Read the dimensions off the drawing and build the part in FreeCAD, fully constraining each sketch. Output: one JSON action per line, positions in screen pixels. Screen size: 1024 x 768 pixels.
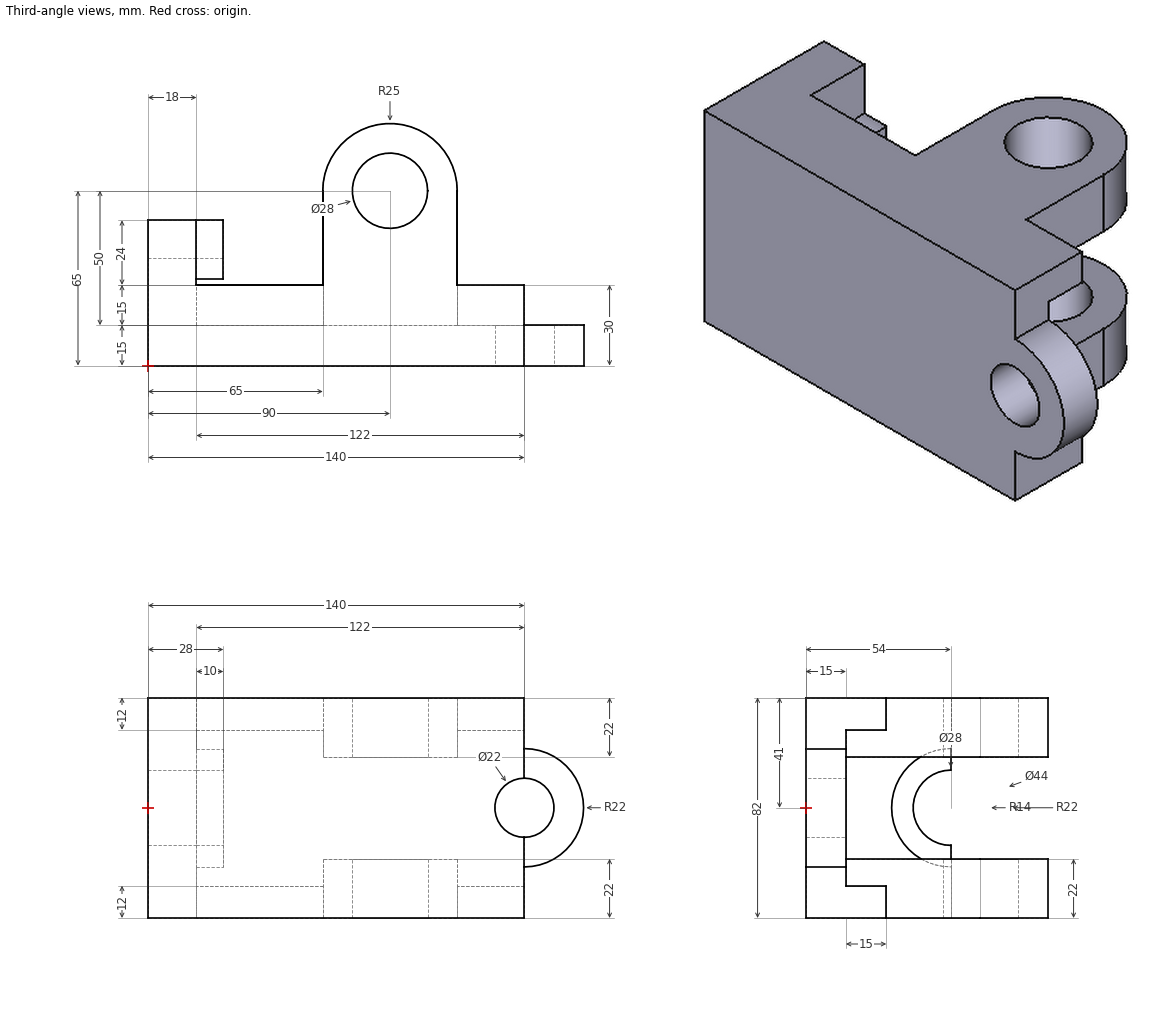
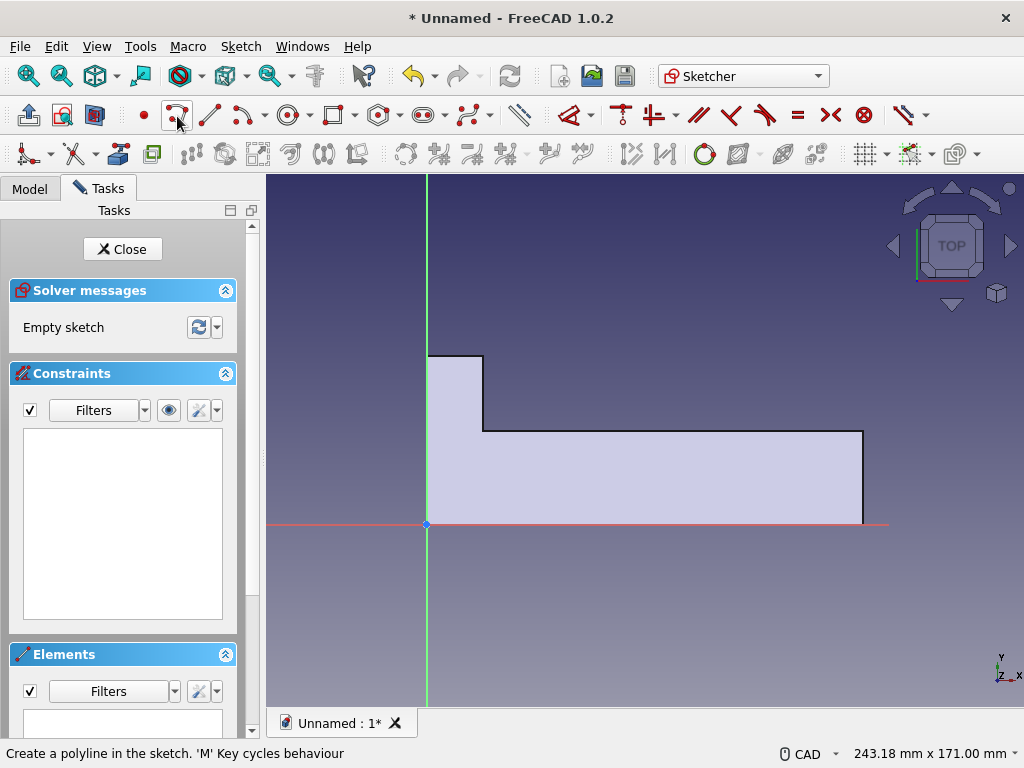
{"action": "left_click", "coordinate": [629, 322]}
{"action": "left_click", "coordinate": [629, 478]}
{"action": "left_click", "coordinate": [785, 478]}
{"action": "left_click", "coordinate": [785, 322]}
{"action": "right_click", "coordinate": [785, 322]}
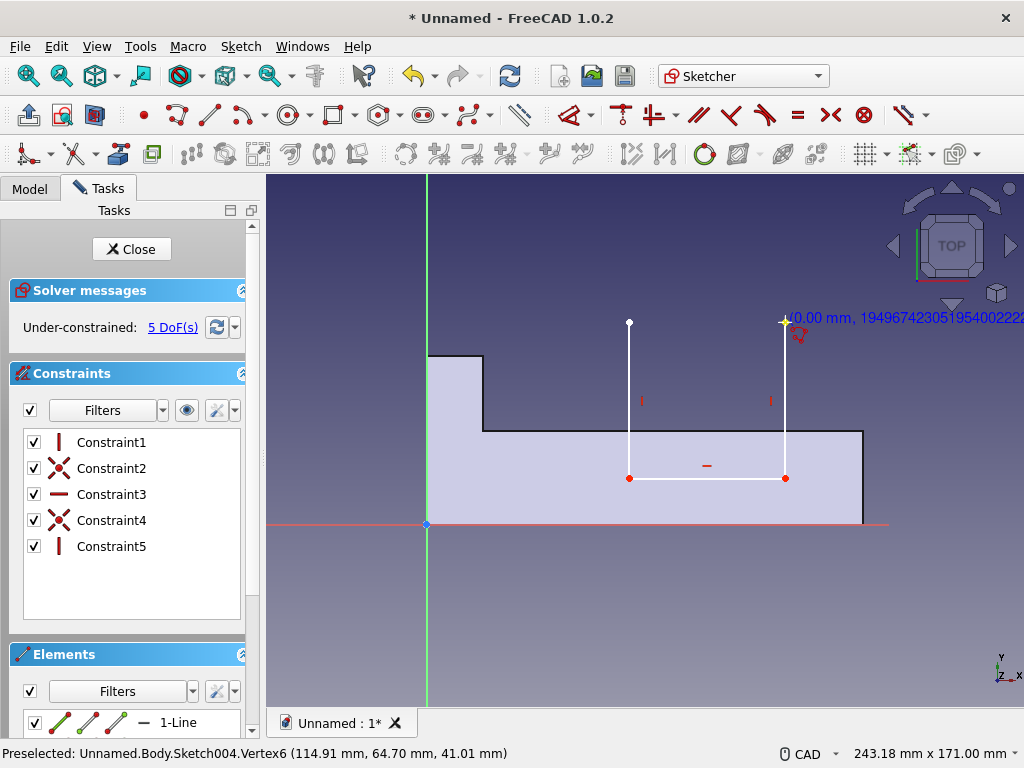
{"action": "key", "text": "g 3 a"}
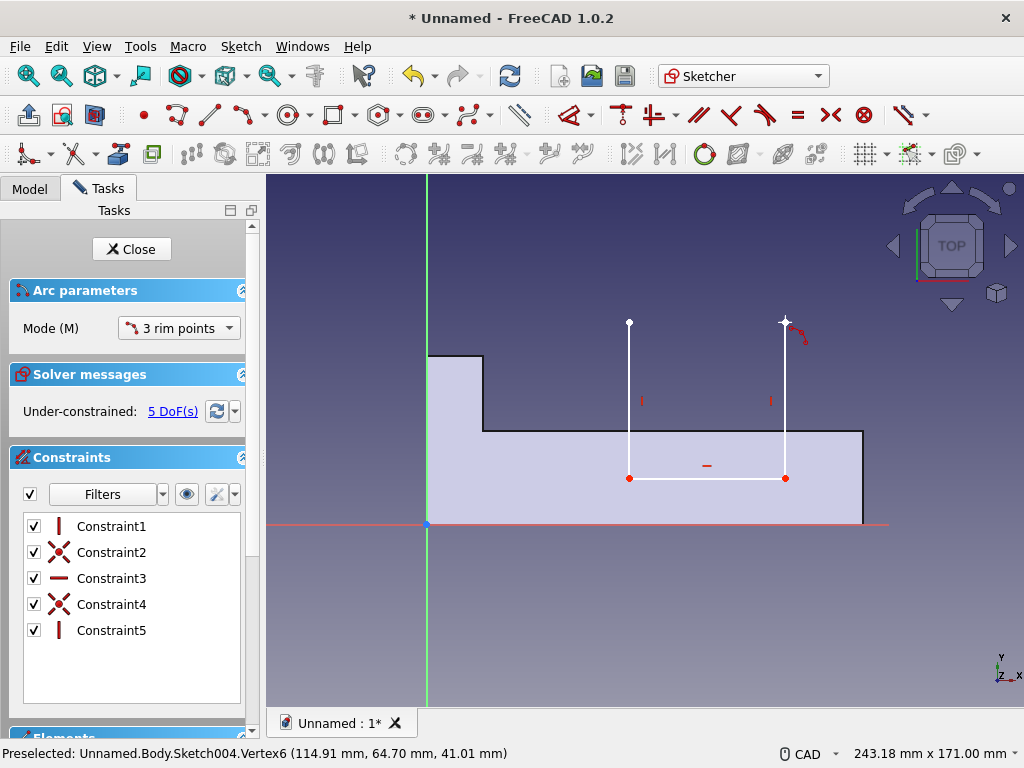
{"action": "left_click", "coordinate": [785, 323]}
{"action": "left_click", "coordinate": [629, 323]}
{"action": "left_click", "coordinate": [707, 244]}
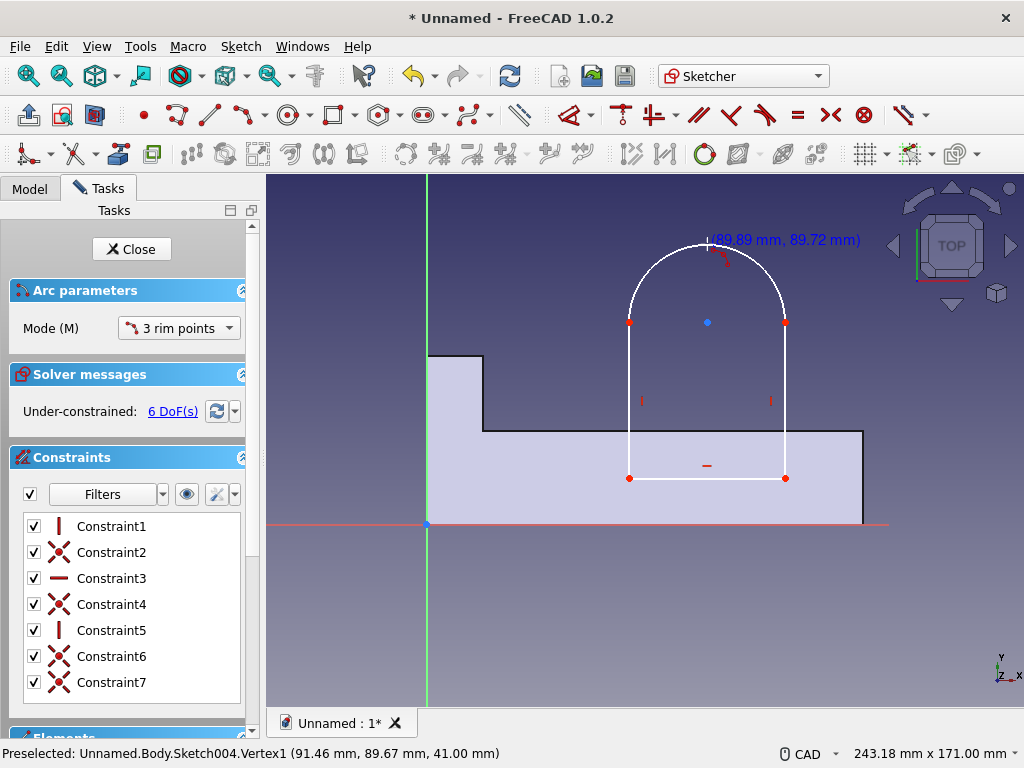
{"action": "left_click", "coordinate": [288, 116]}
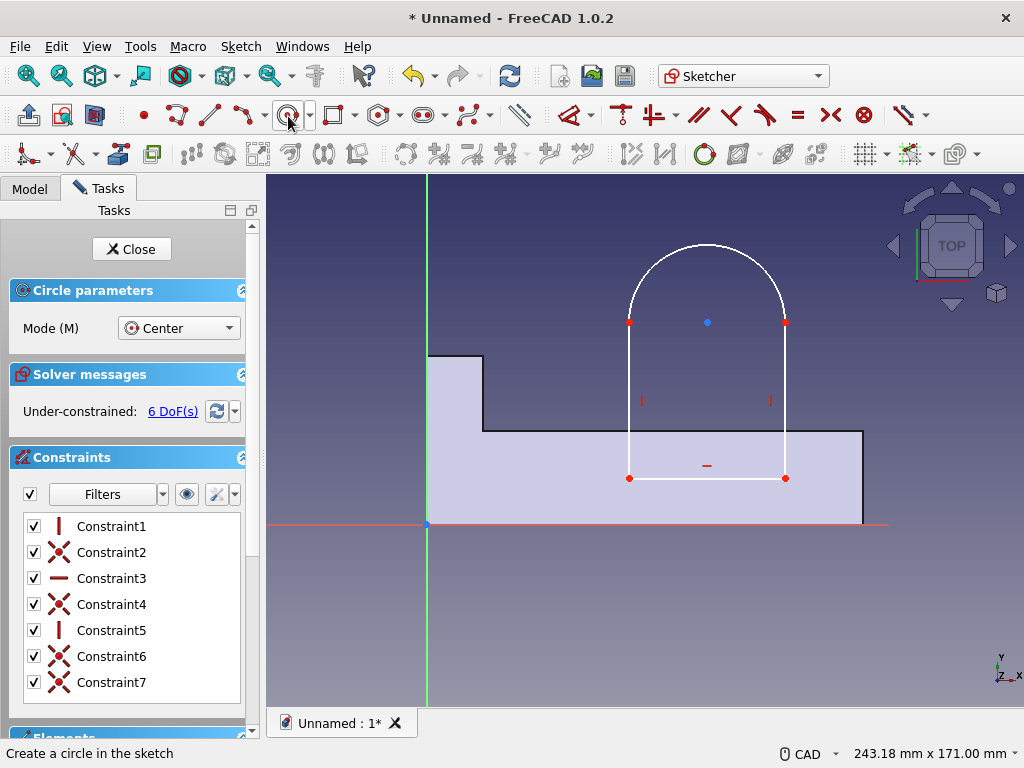
{"action": "left_click", "coordinate": [707, 322]}
{"action": "left_click", "coordinate": [738, 291]}
{"action": "key", "text": "Escape"}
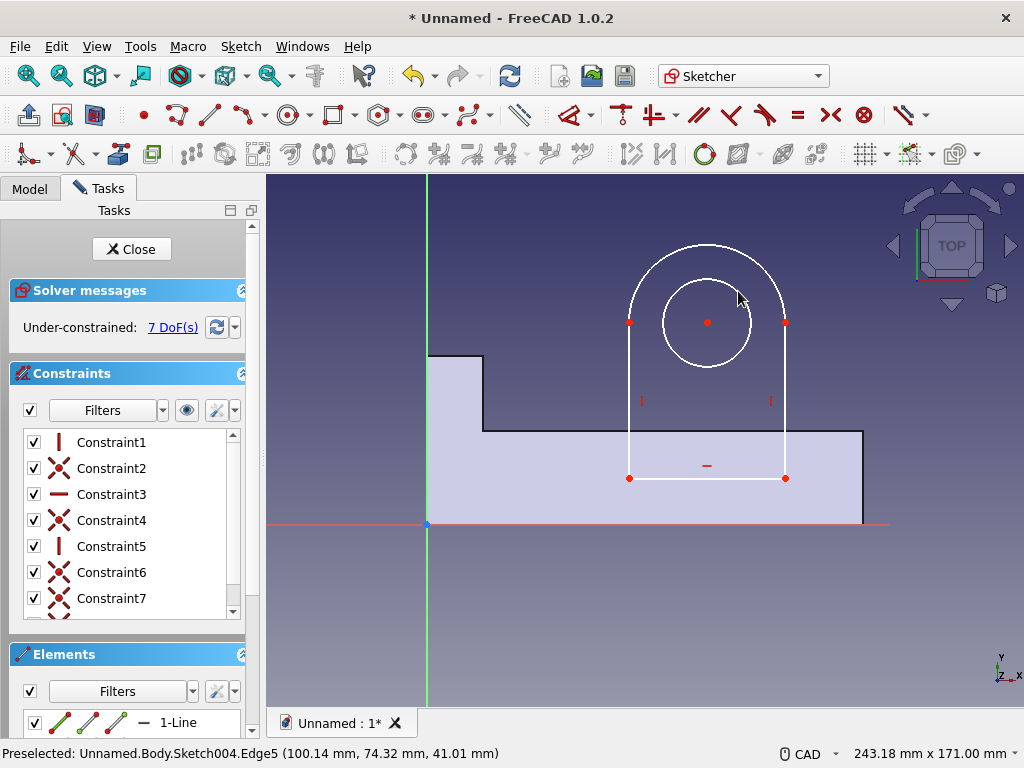
{"action": "left_click", "coordinate": [629, 370]}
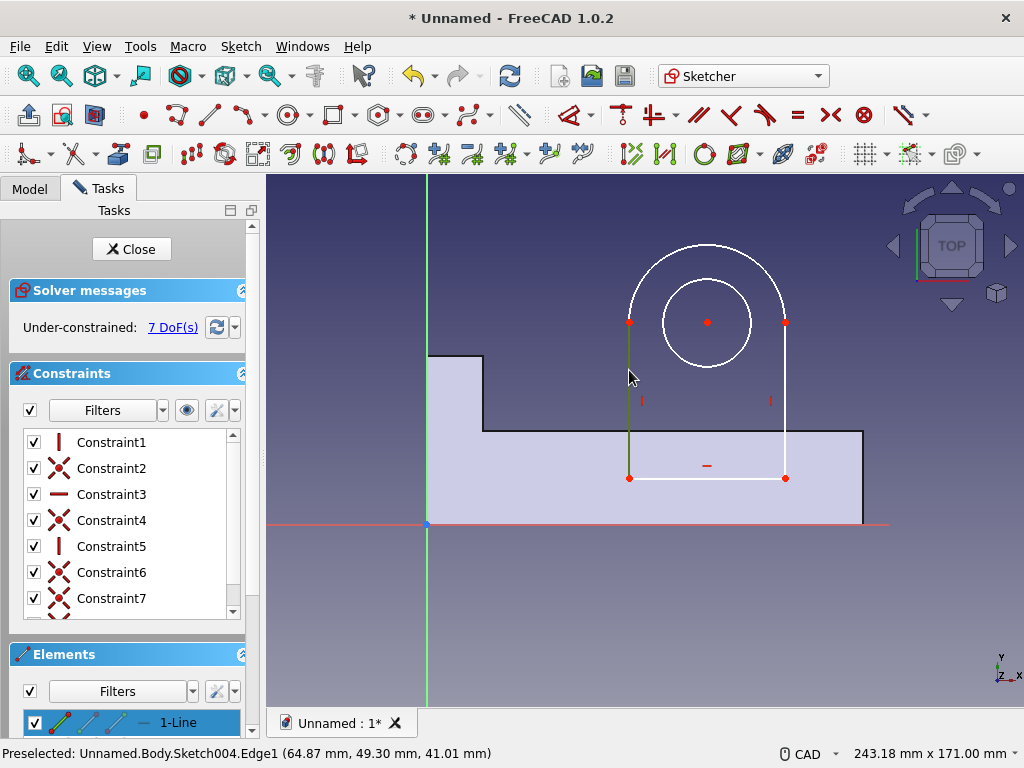
{"action": "left_click", "coordinate": [753, 260]}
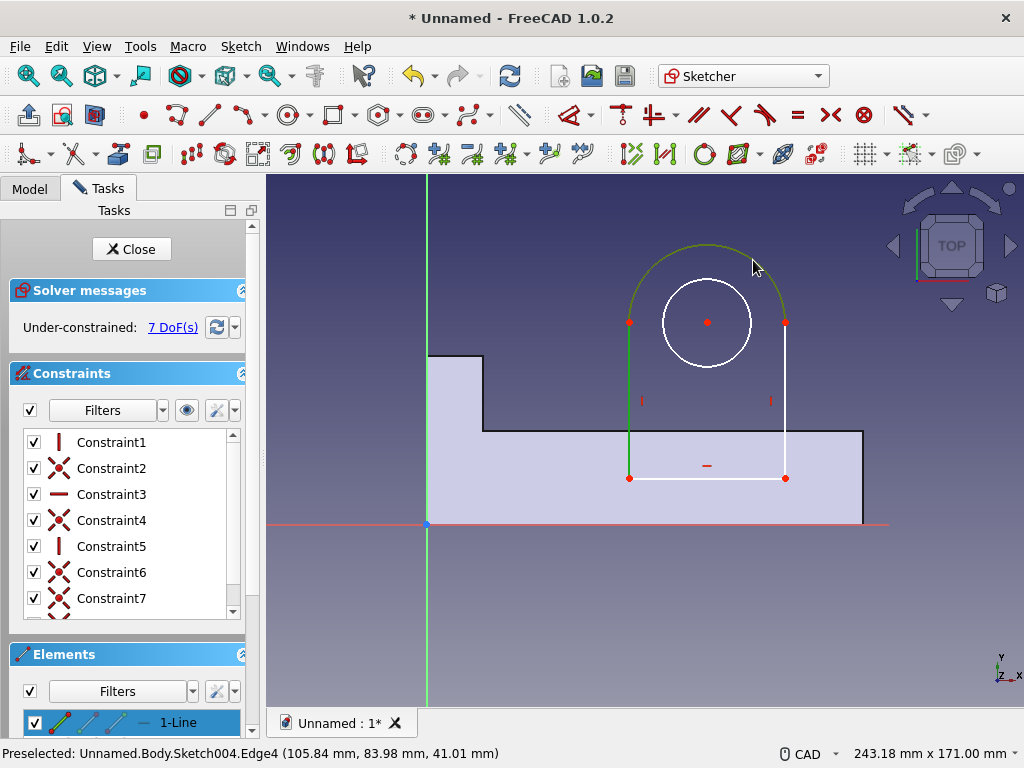
{"action": "key", "text": "t"}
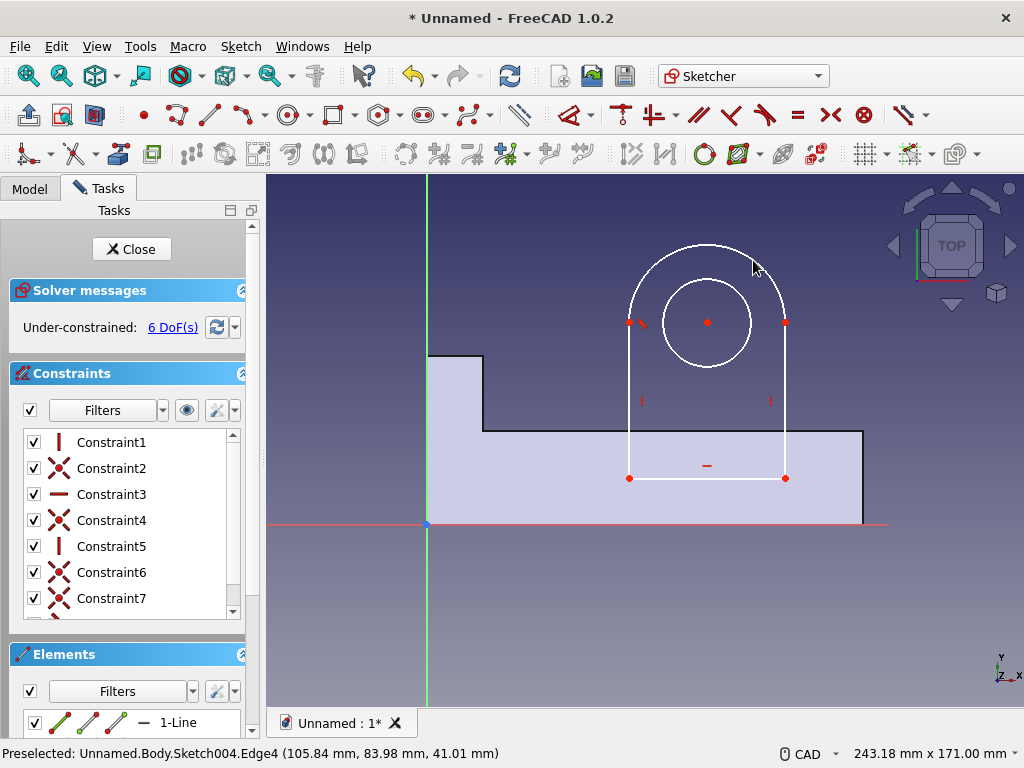
{"action": "left_click", "coordinate": [785, 432]}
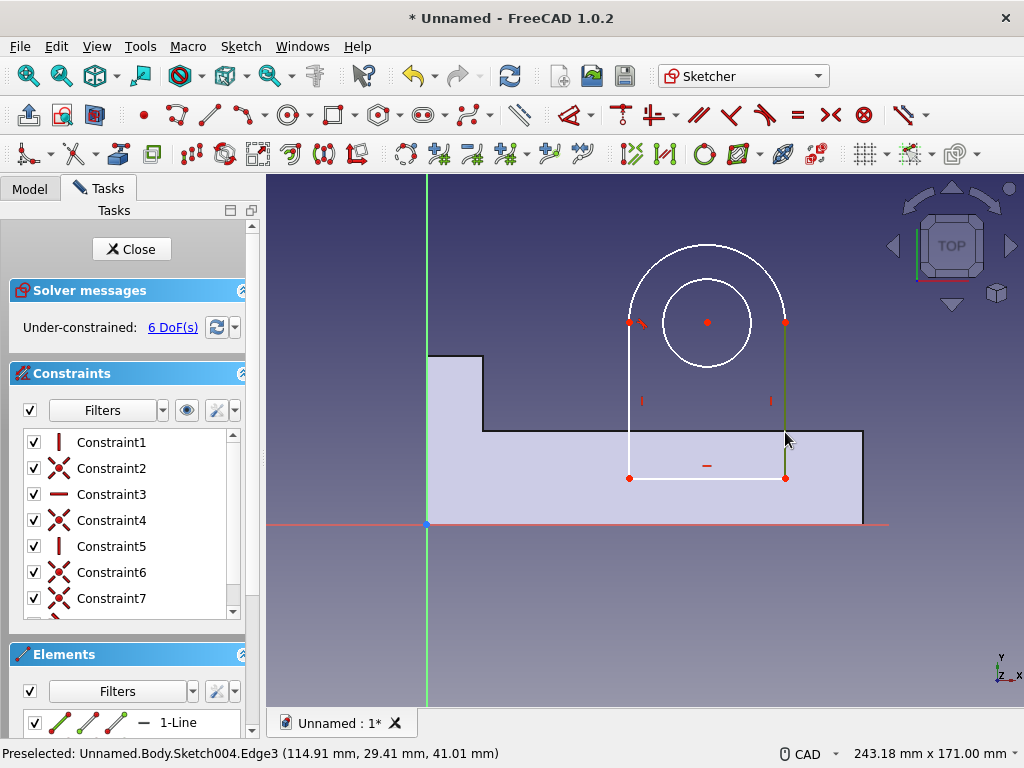
{"action": "left_click", "coordinate": [753, 260]}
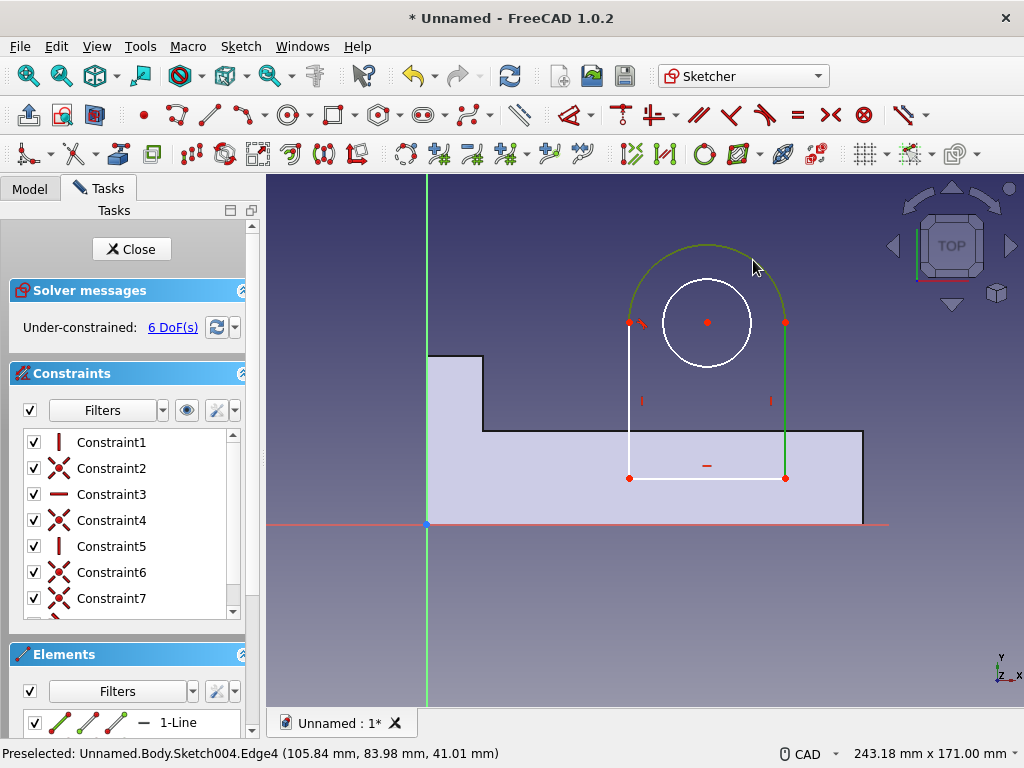
{"action": "key", "text": "t"}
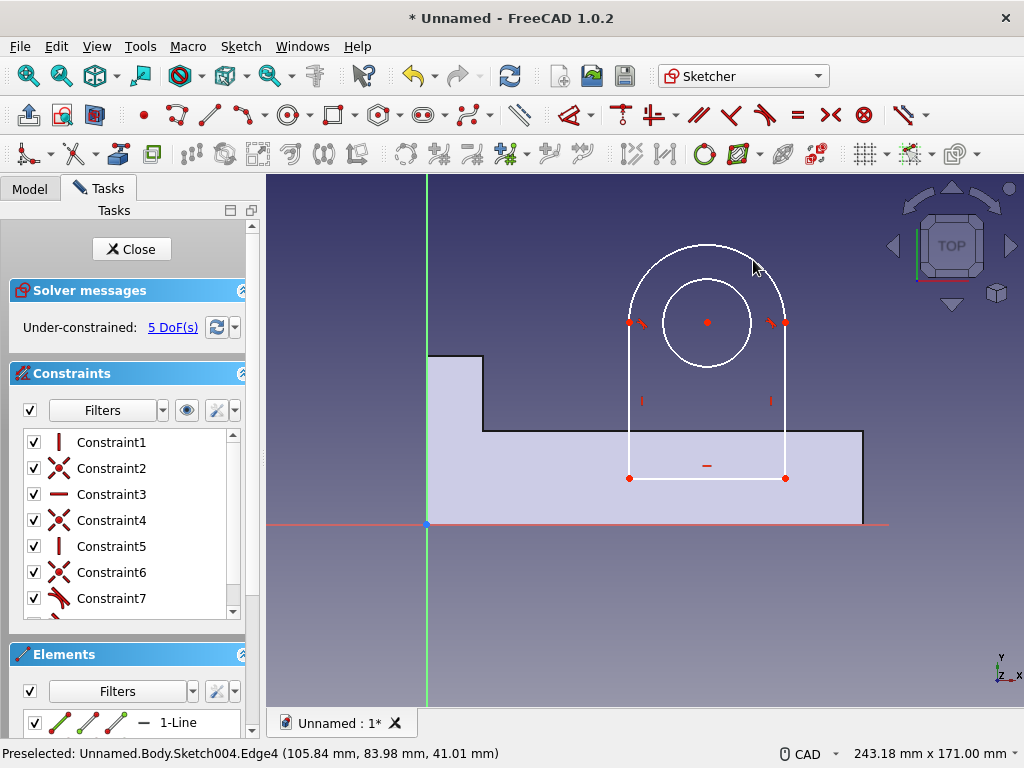
{"action": "left_click", "coordinate": [568, 116]}